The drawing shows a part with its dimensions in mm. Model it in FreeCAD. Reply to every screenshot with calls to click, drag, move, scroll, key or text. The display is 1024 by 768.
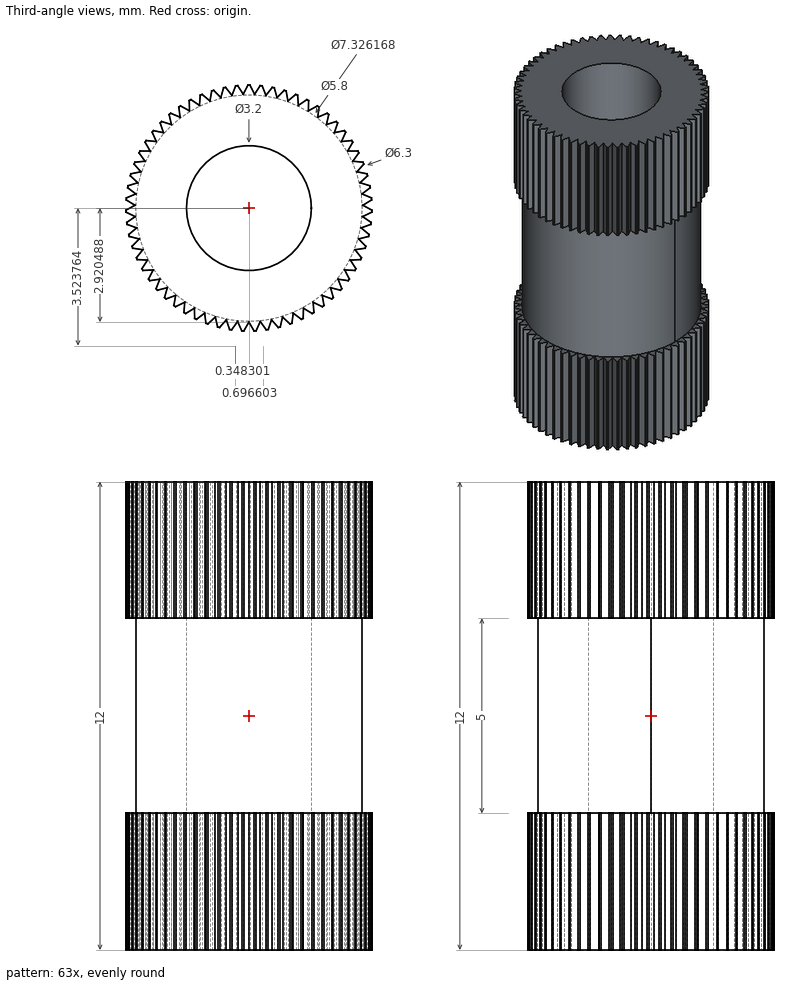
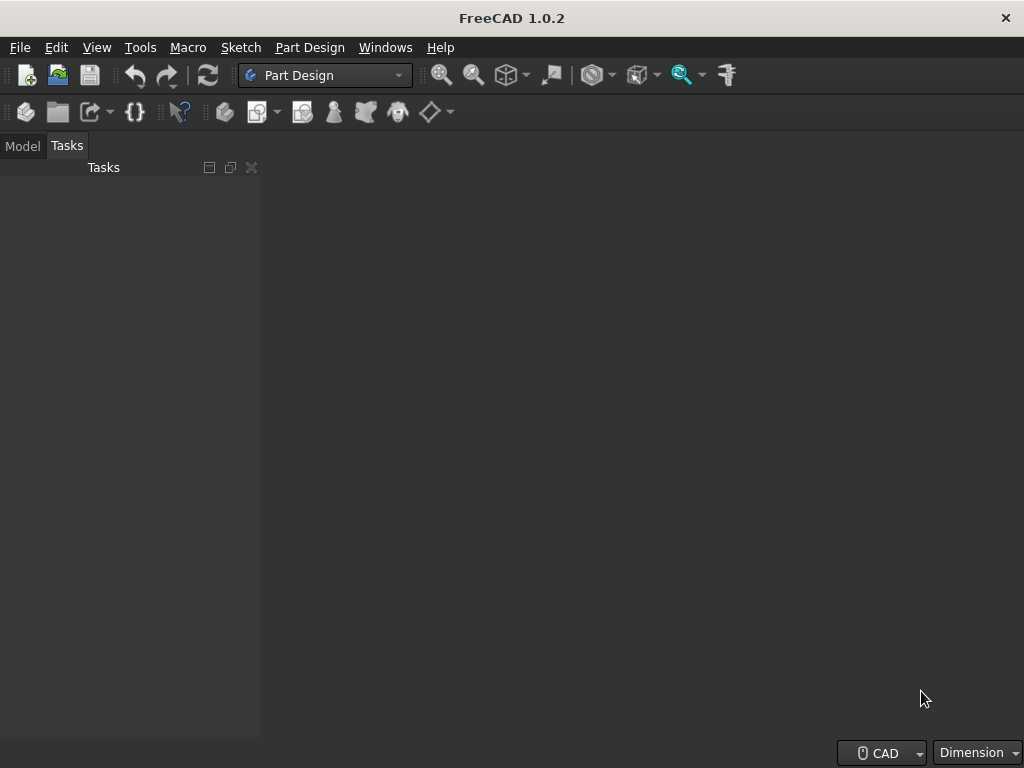
click(168, 76)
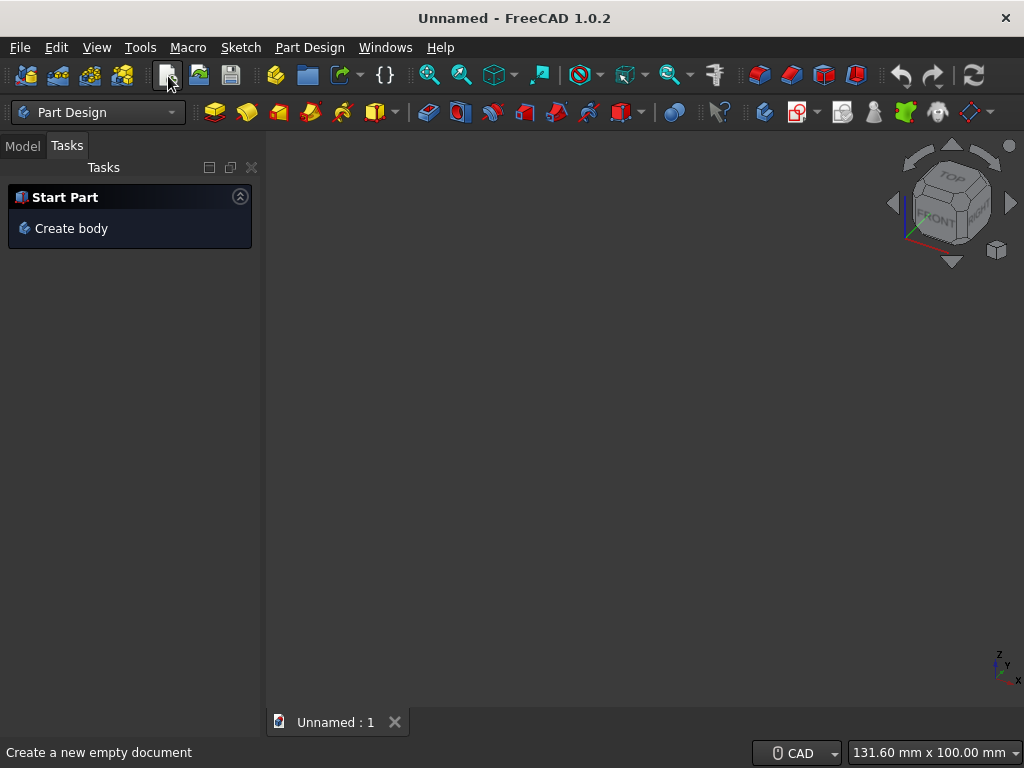
click(798, 112)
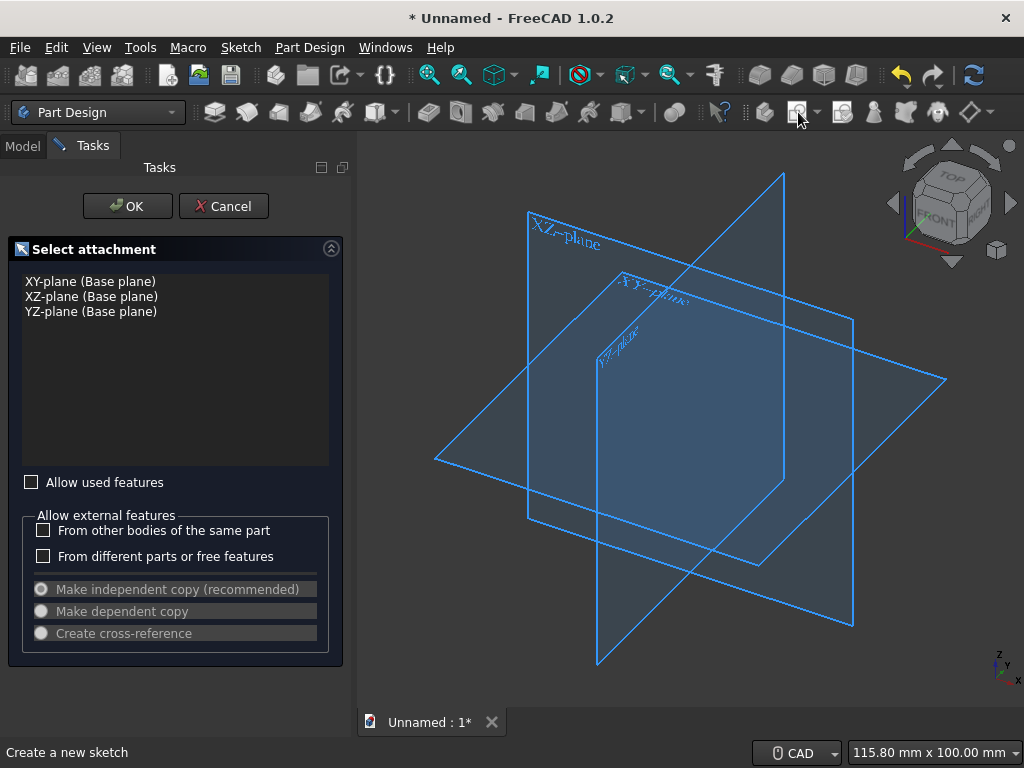
click(82, 282)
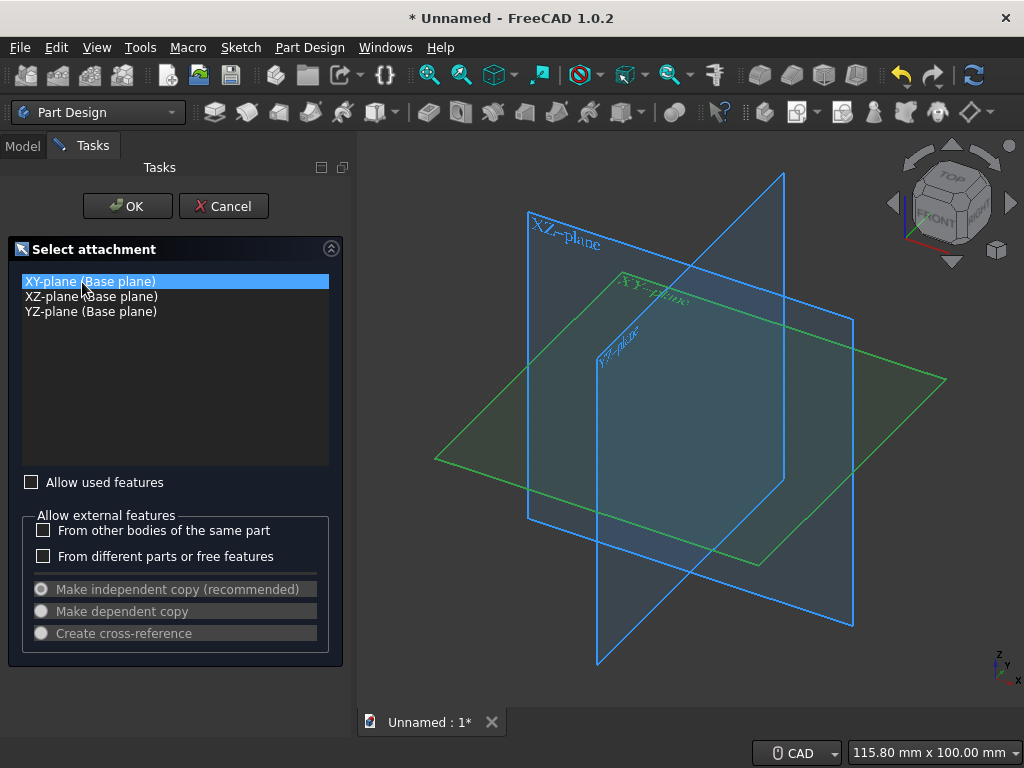
click(128, 206)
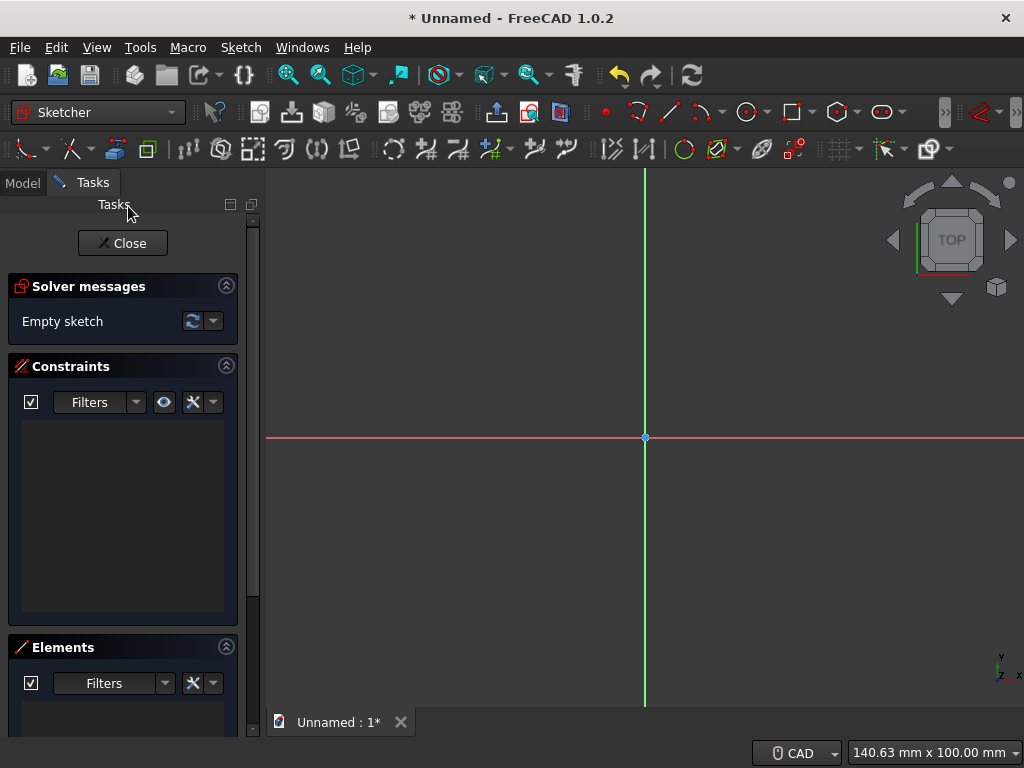
scroll(652, 438, up, 12)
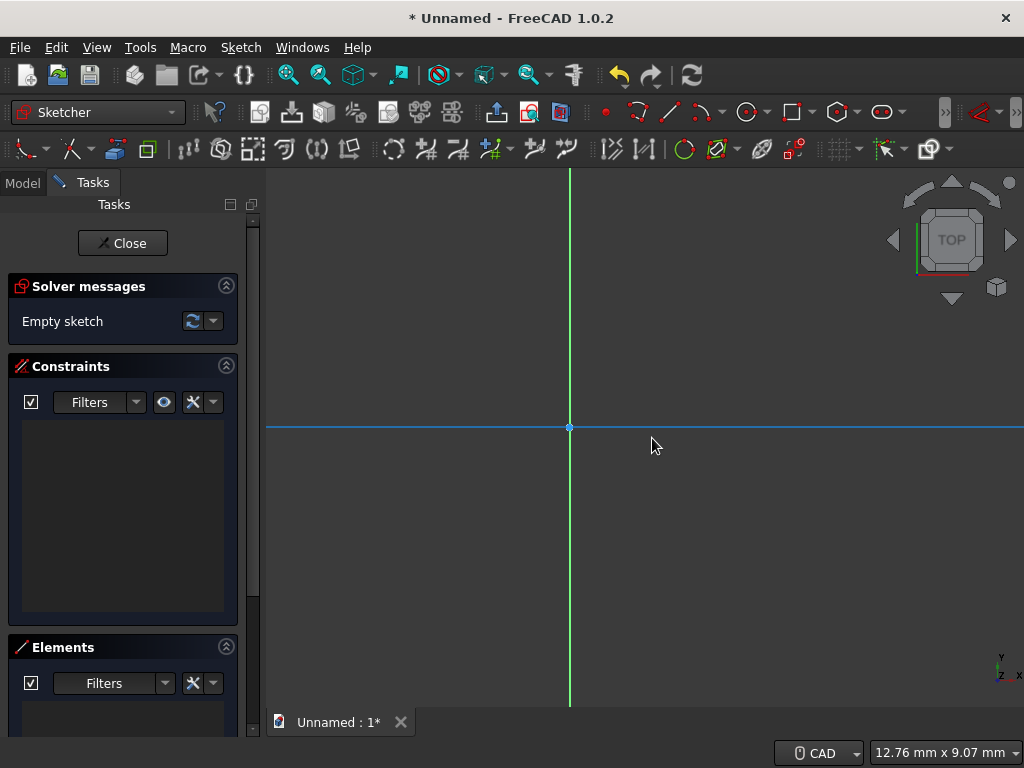
click(748, 112)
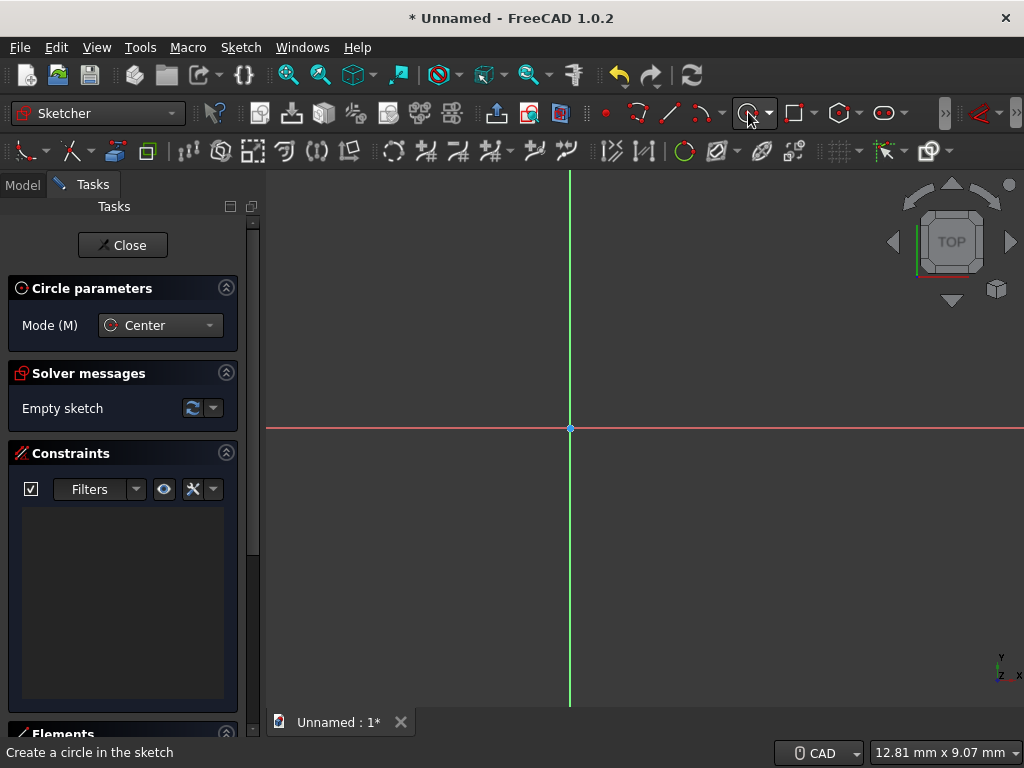
click(570, 428)
click(702, 297)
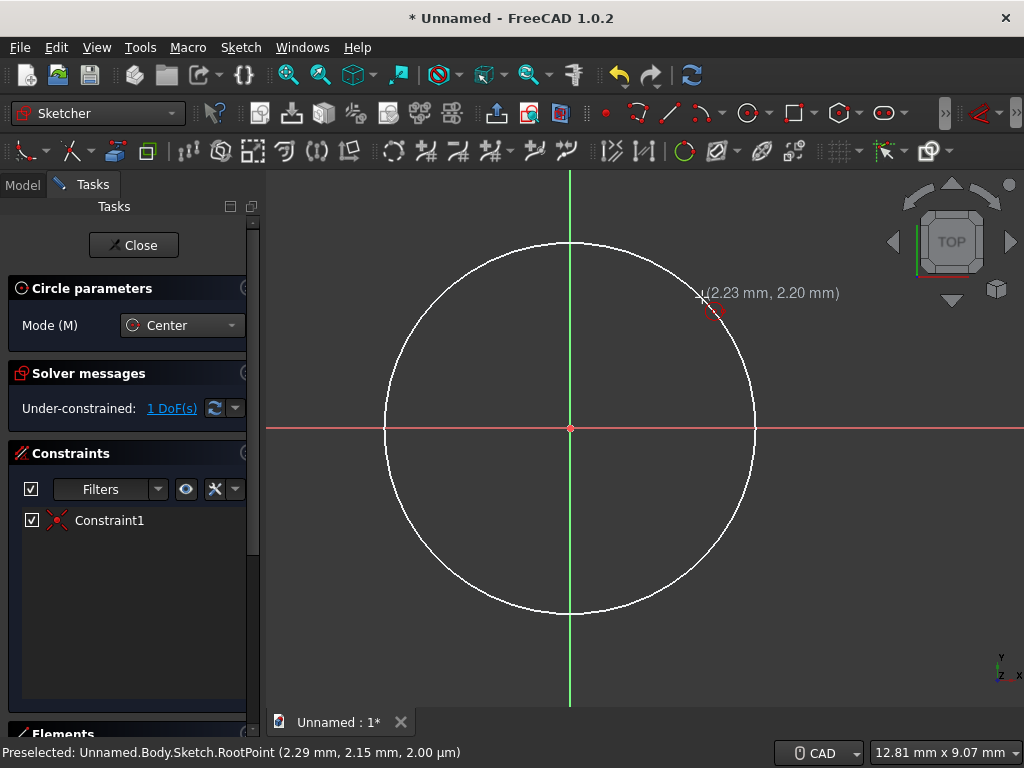
click(570, 428)
click(637, 362)
key(Escape)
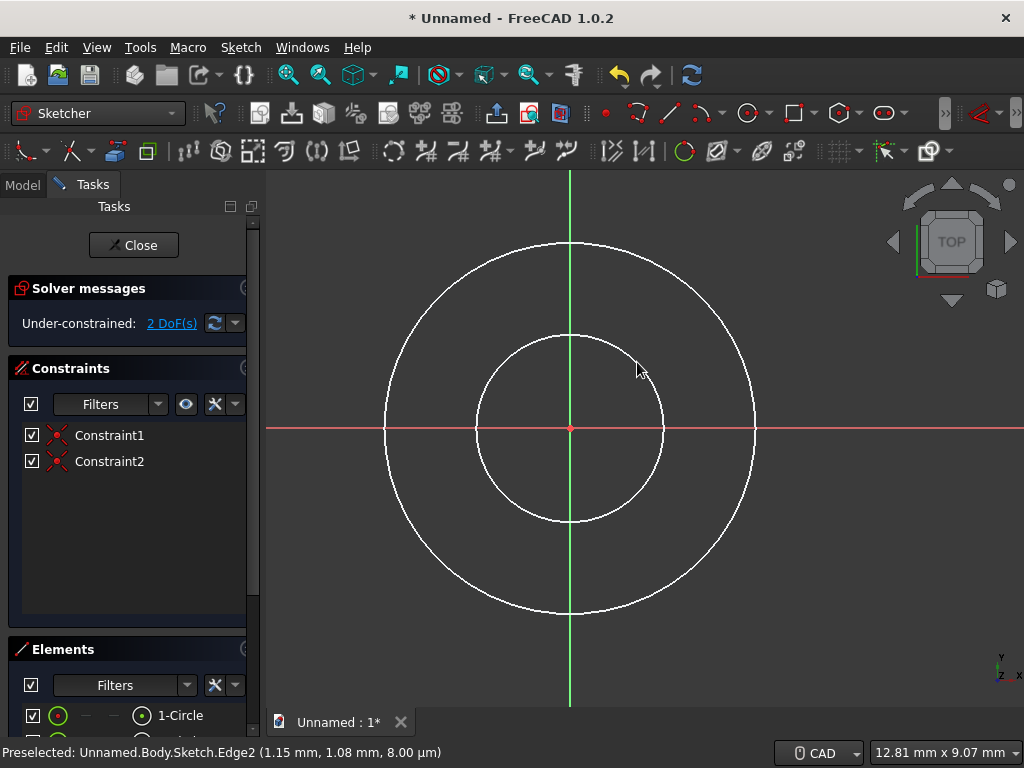
click(980, 114)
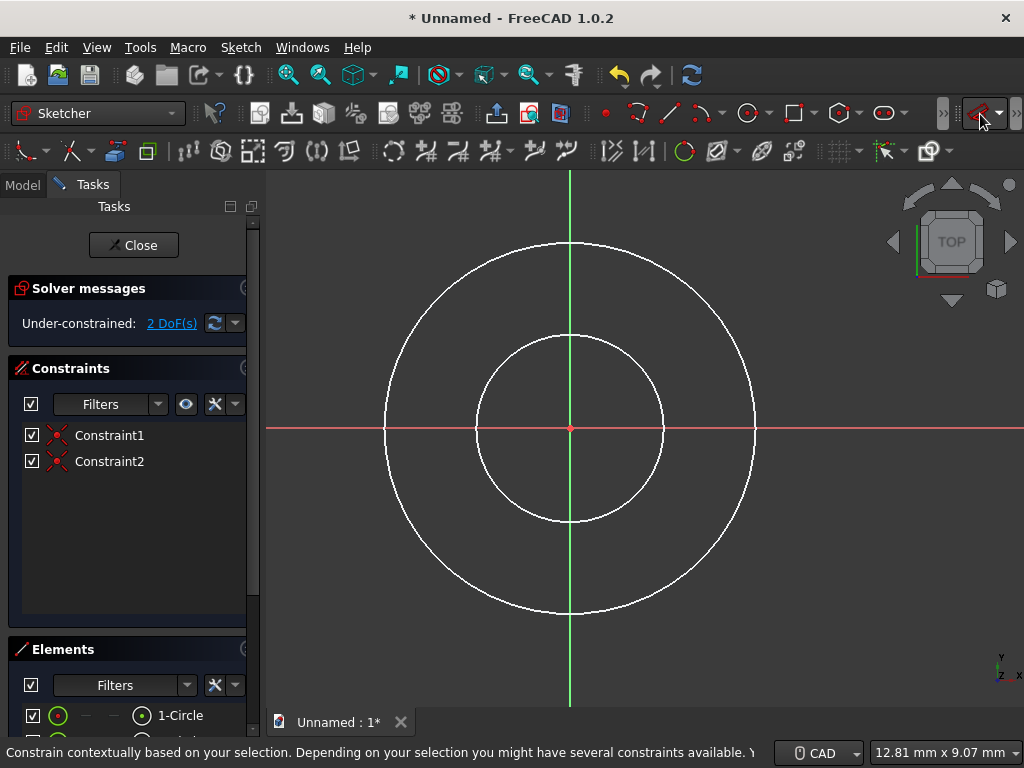
click(701, 297)
click(724, 274)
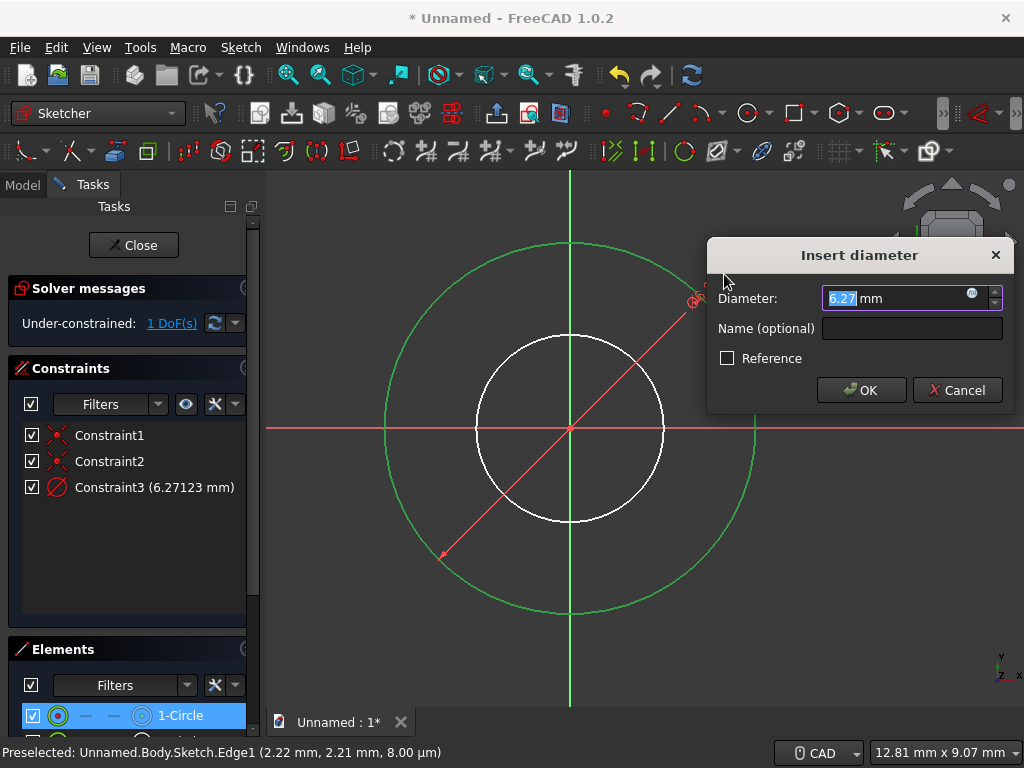
text(6.3)
key(Return)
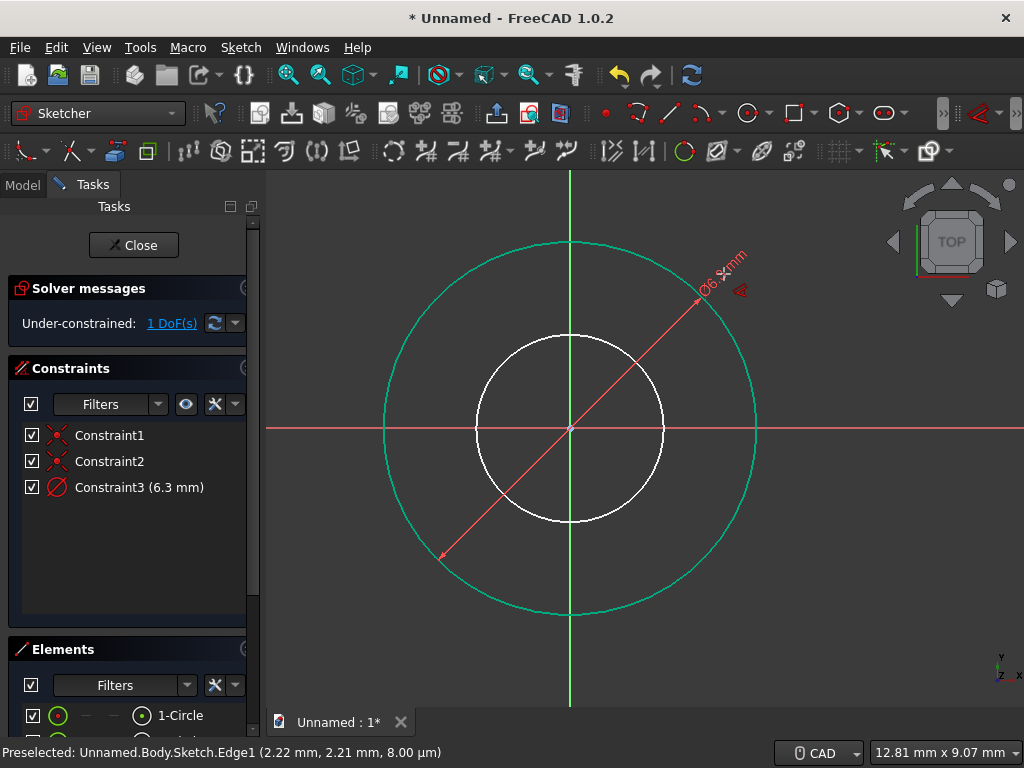
click(636, 362)
click(659, 339)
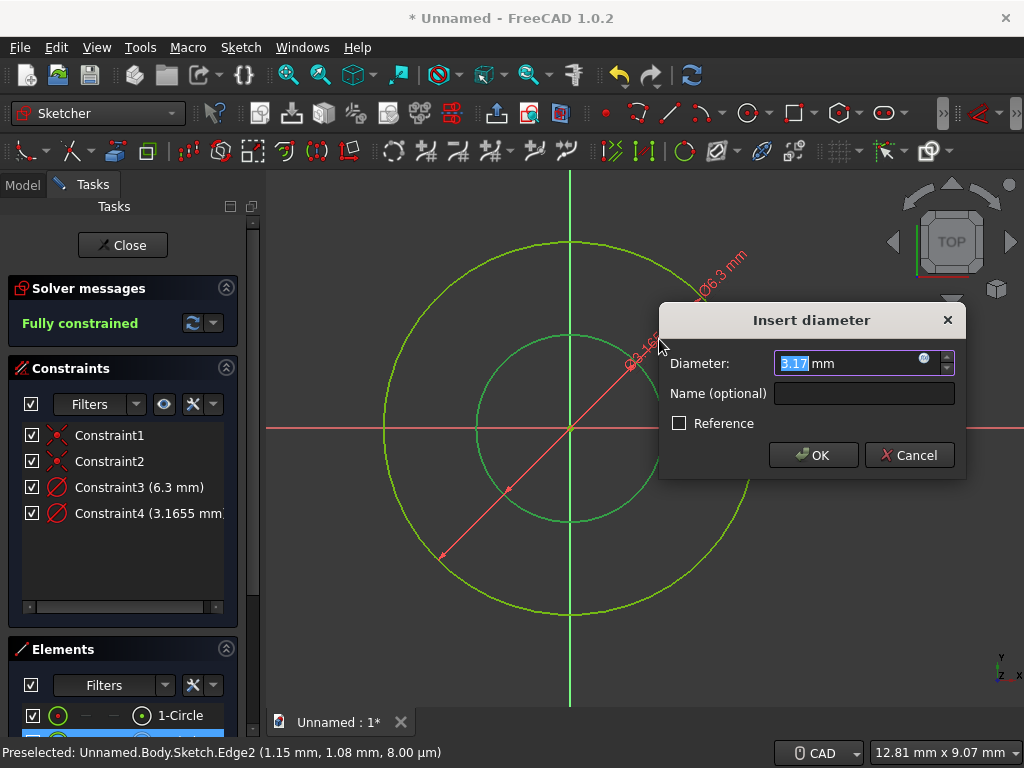
text(3.2)
key(Return)
key(Escape)